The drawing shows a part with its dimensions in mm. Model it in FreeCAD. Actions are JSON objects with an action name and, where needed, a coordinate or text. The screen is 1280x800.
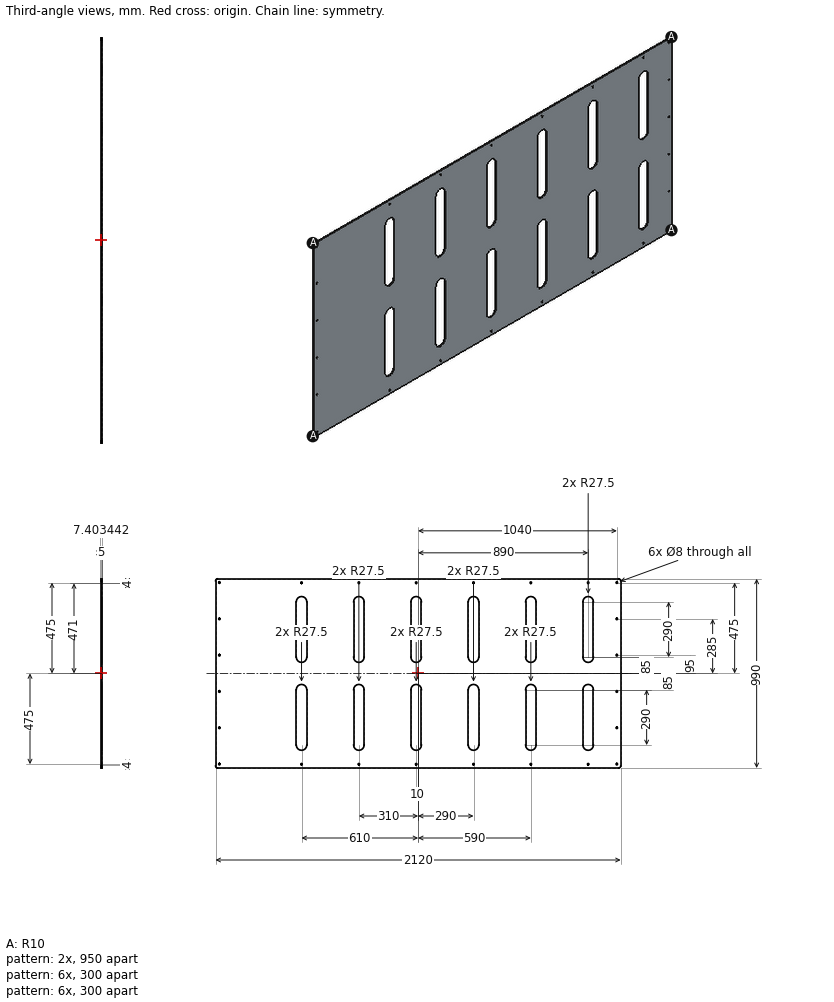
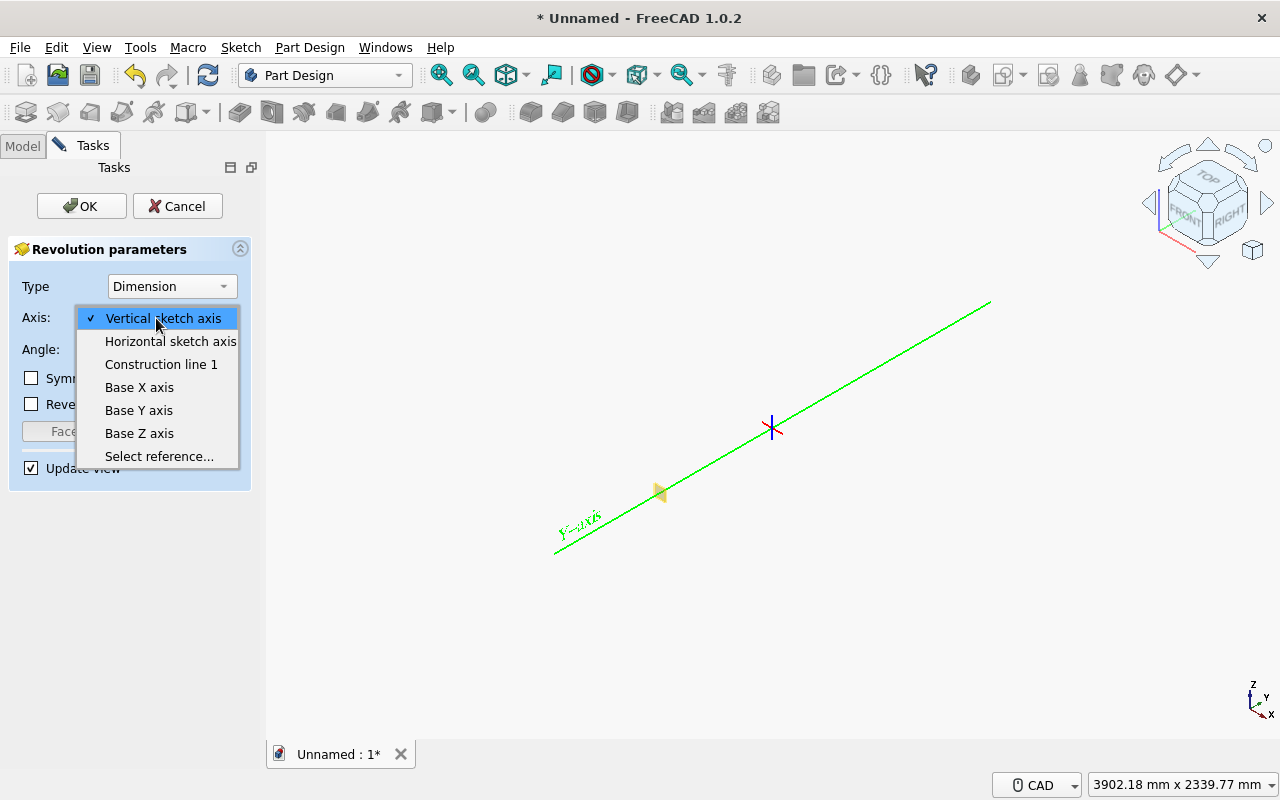
{"action": "left_click", "coordinate": [156, 364]}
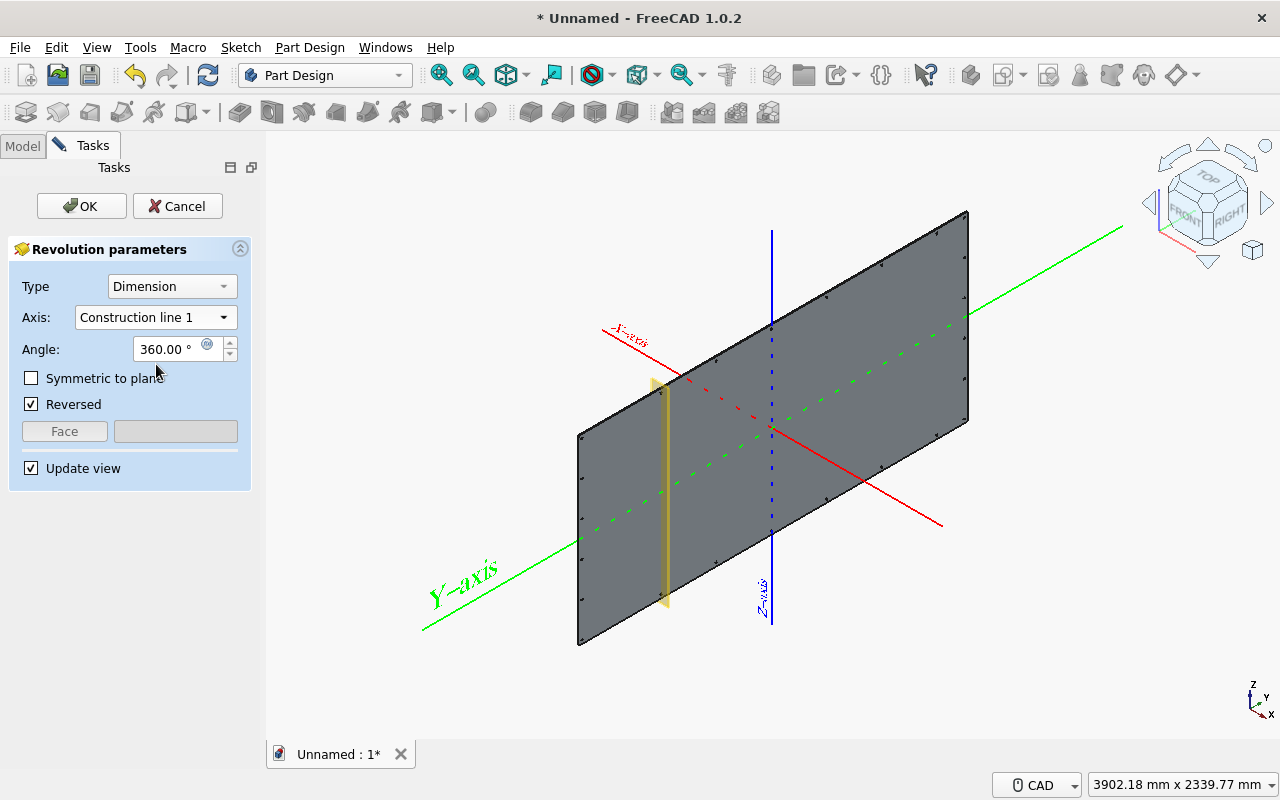
{"action": "left_click", "coordinate": [82, 206]}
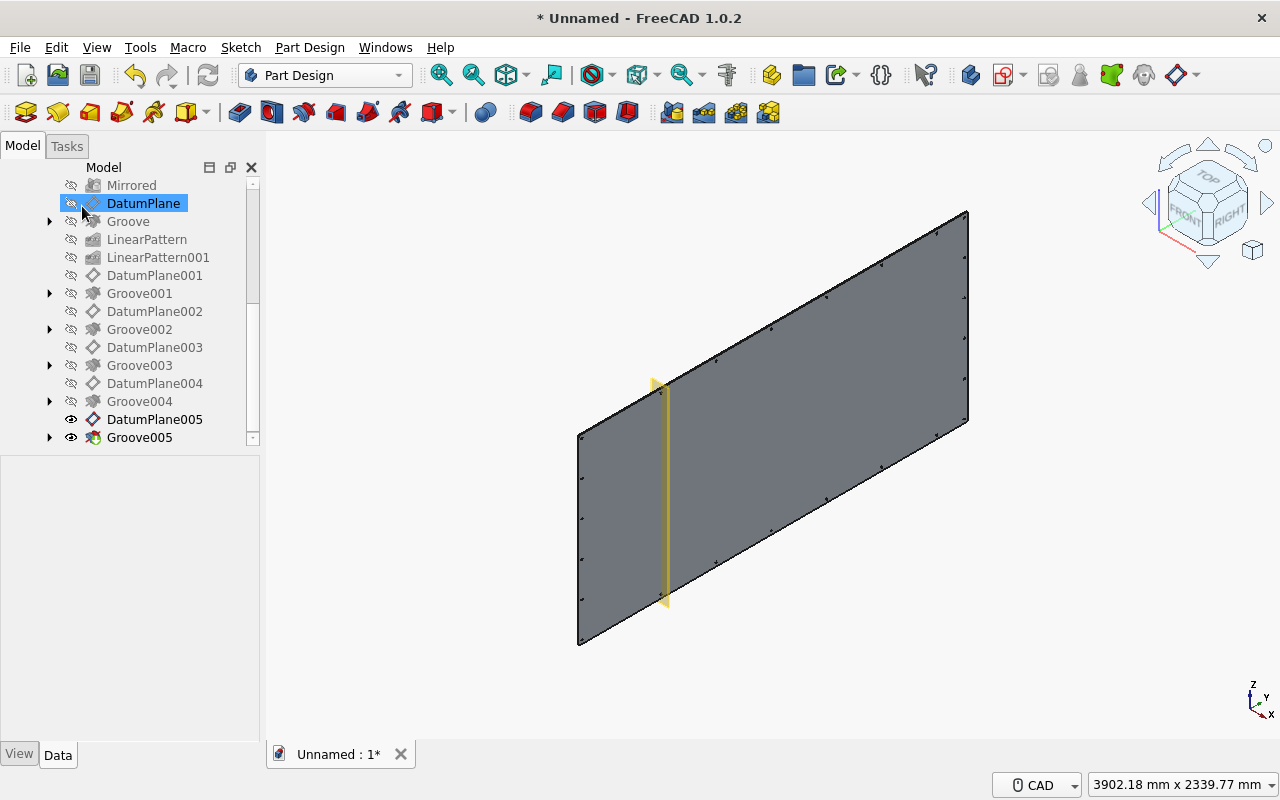
{"action": "left_click", "coordinate": [116, 419]}
{"action": "key", "text": "space"}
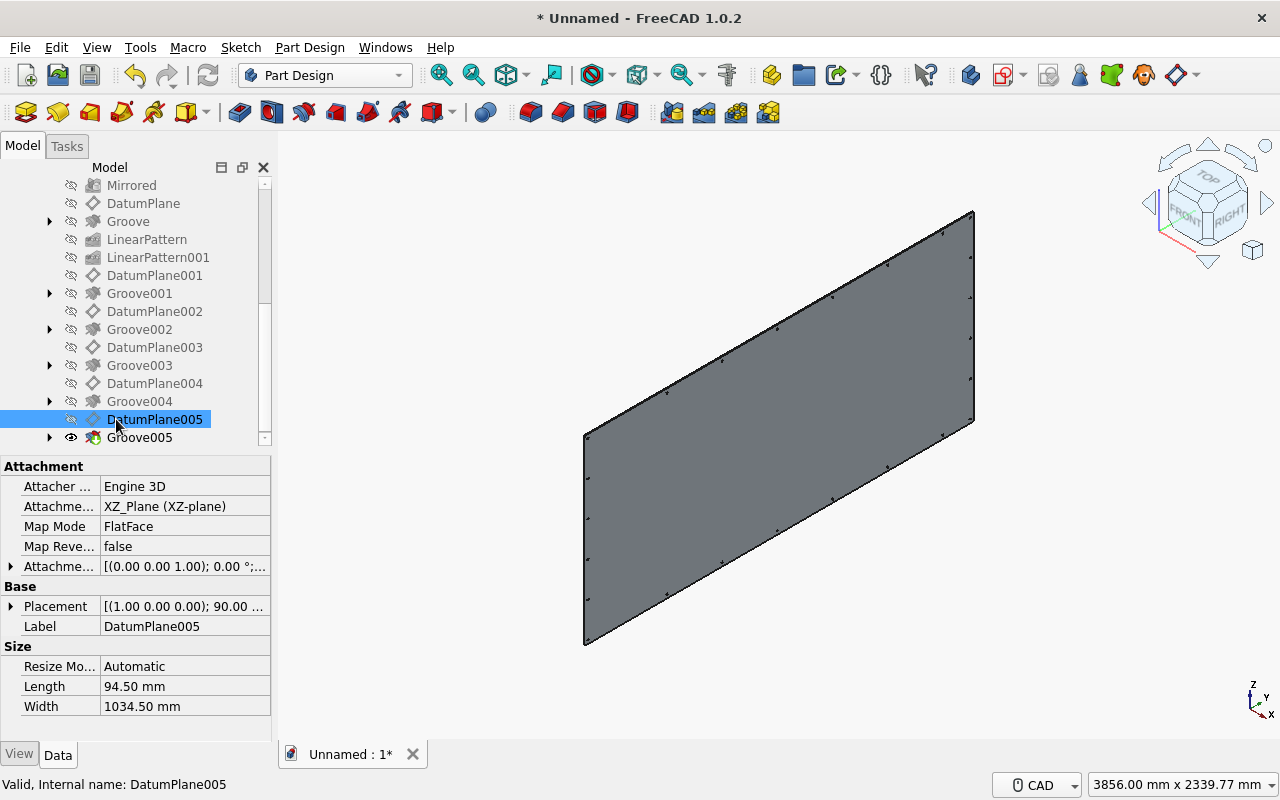
{"action": "left_click", "coordinate": [835, 396]}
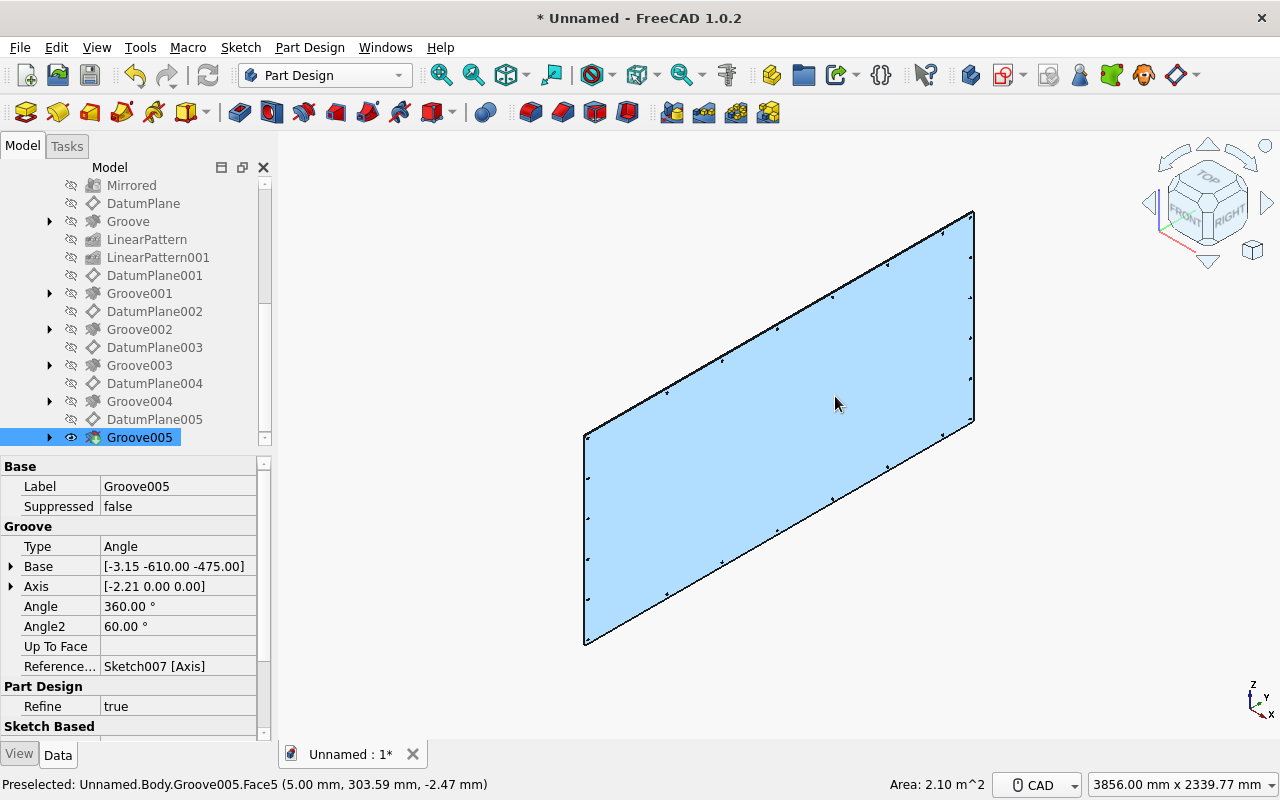
{"action": "left_click", "coordinate": [1004, 76]}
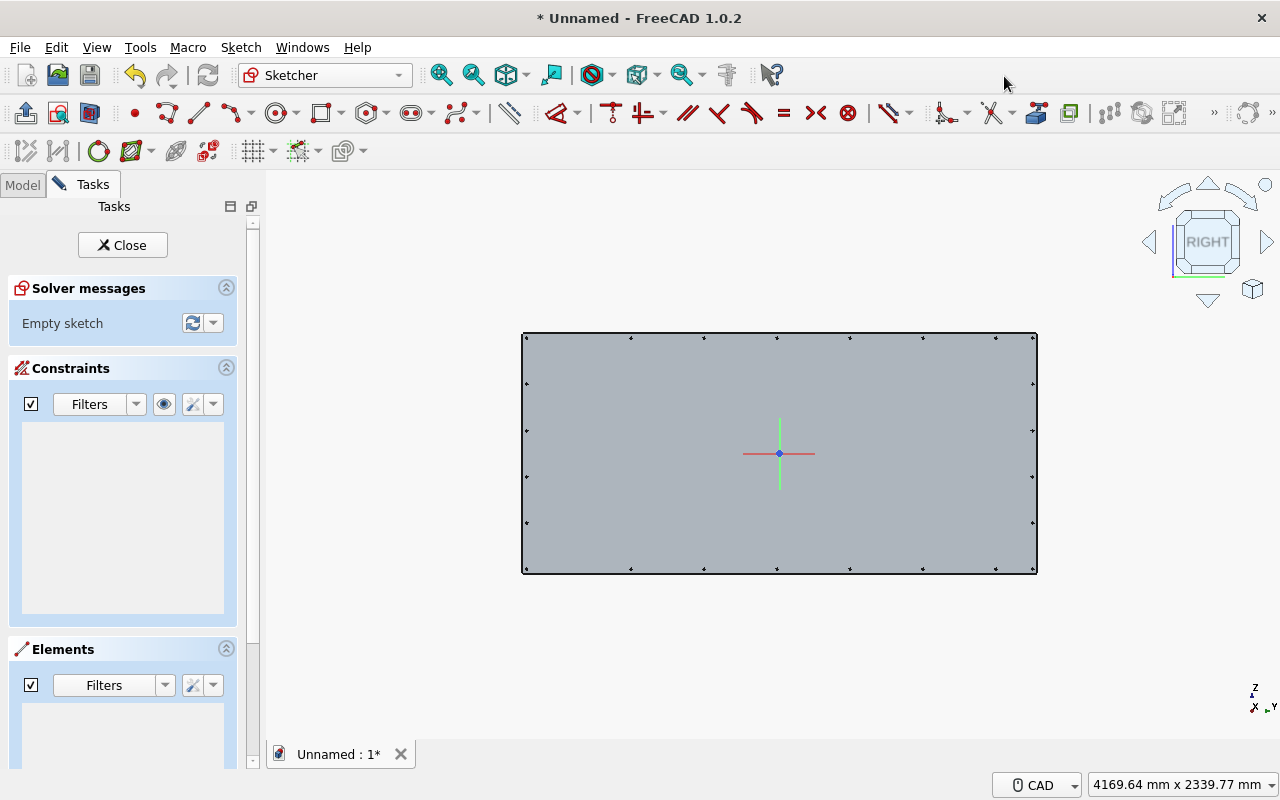
{"action": "scroll", "coordinate": [1091, 379], "scroll_direction": "up", "scroll_amount": 7}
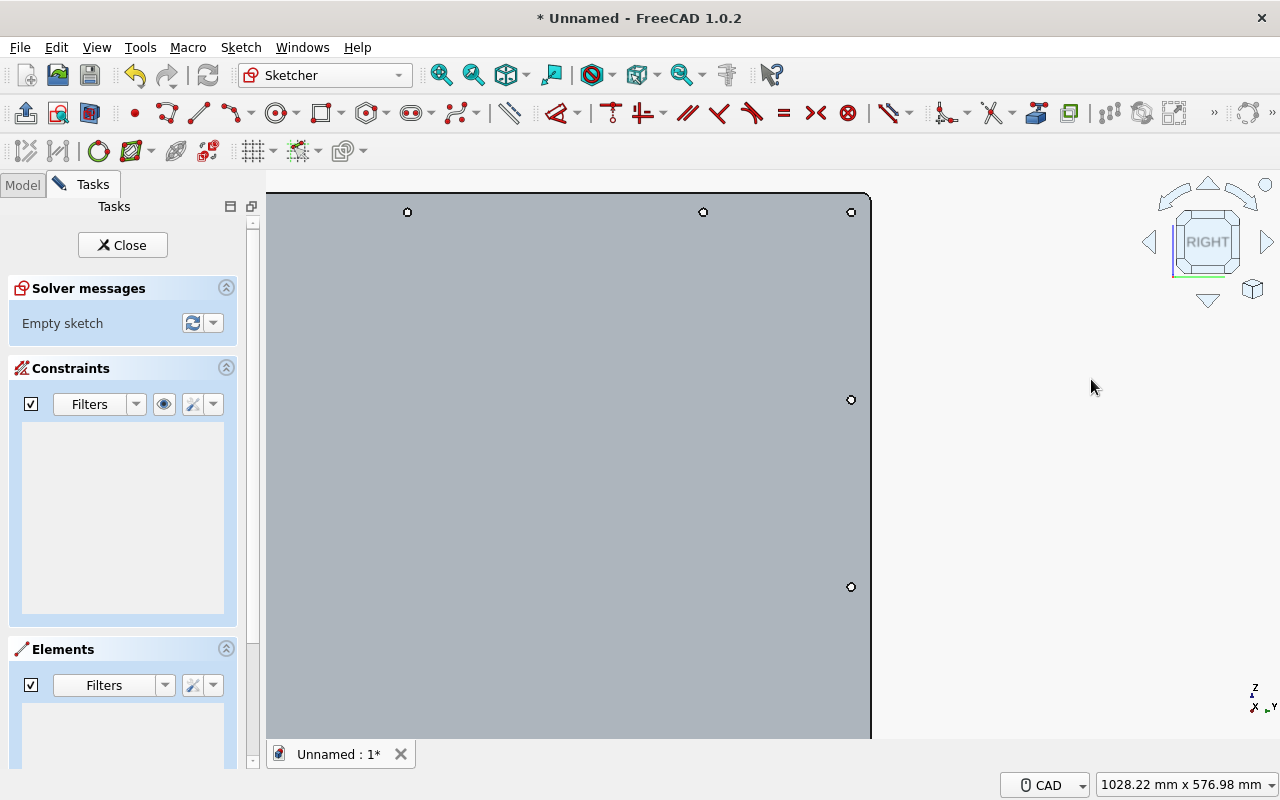
{"action": "left_click", "coordinate": [412, 114]}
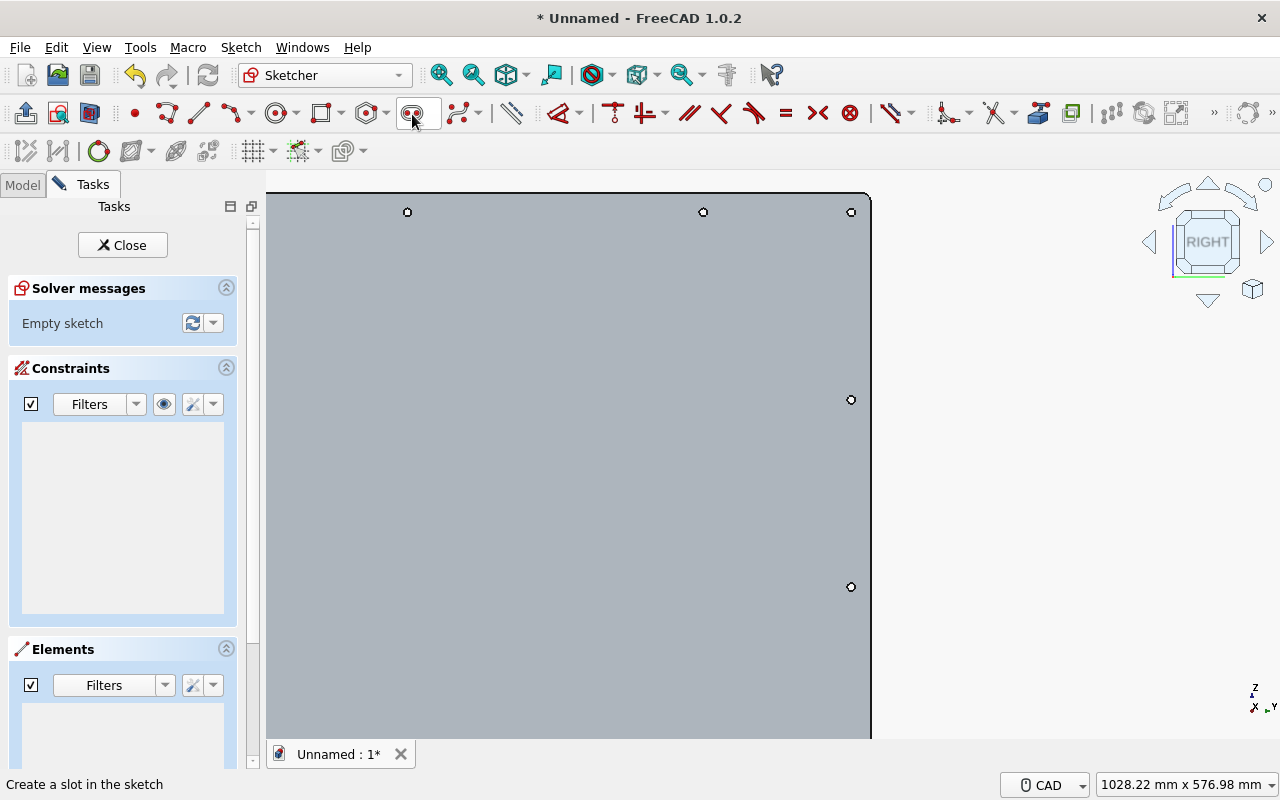
{"action": "left_click", "coordinate": [703, 597]}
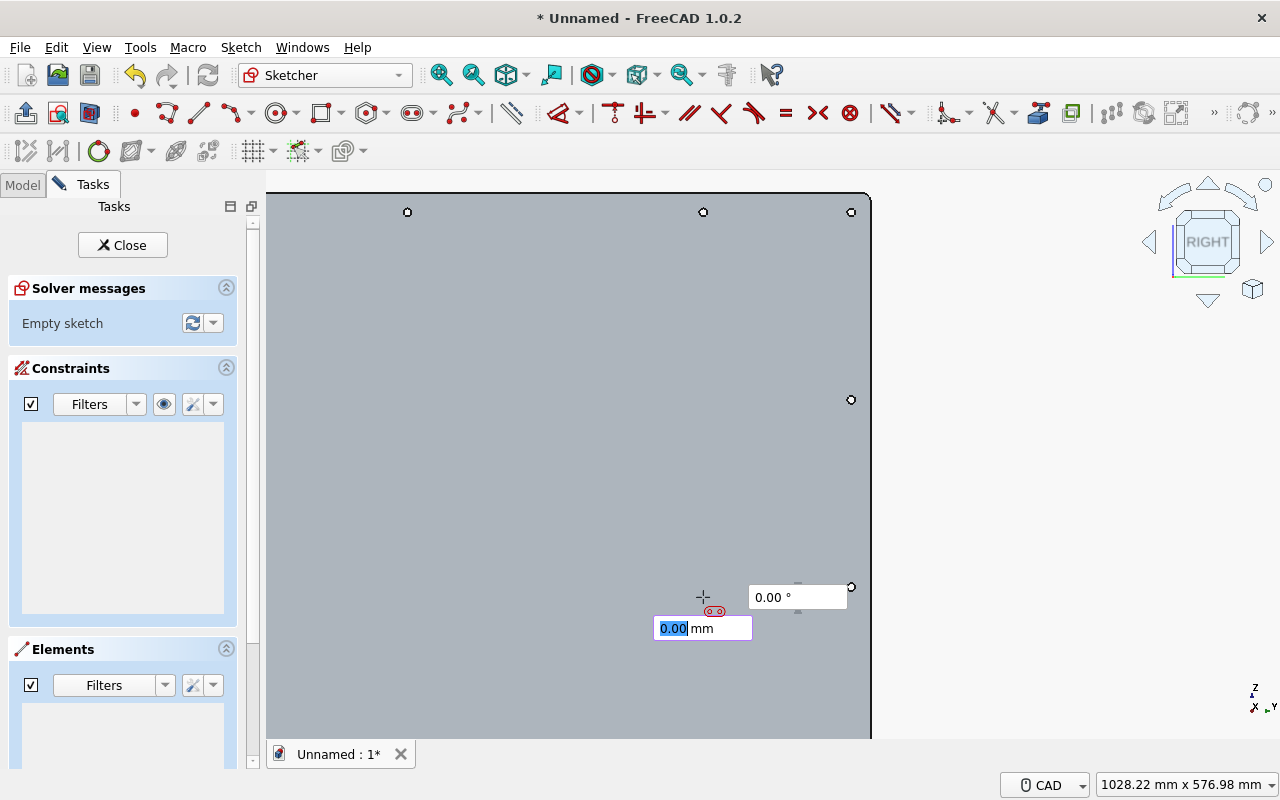
{"action": "left_click", "coordinate": [703, 311]}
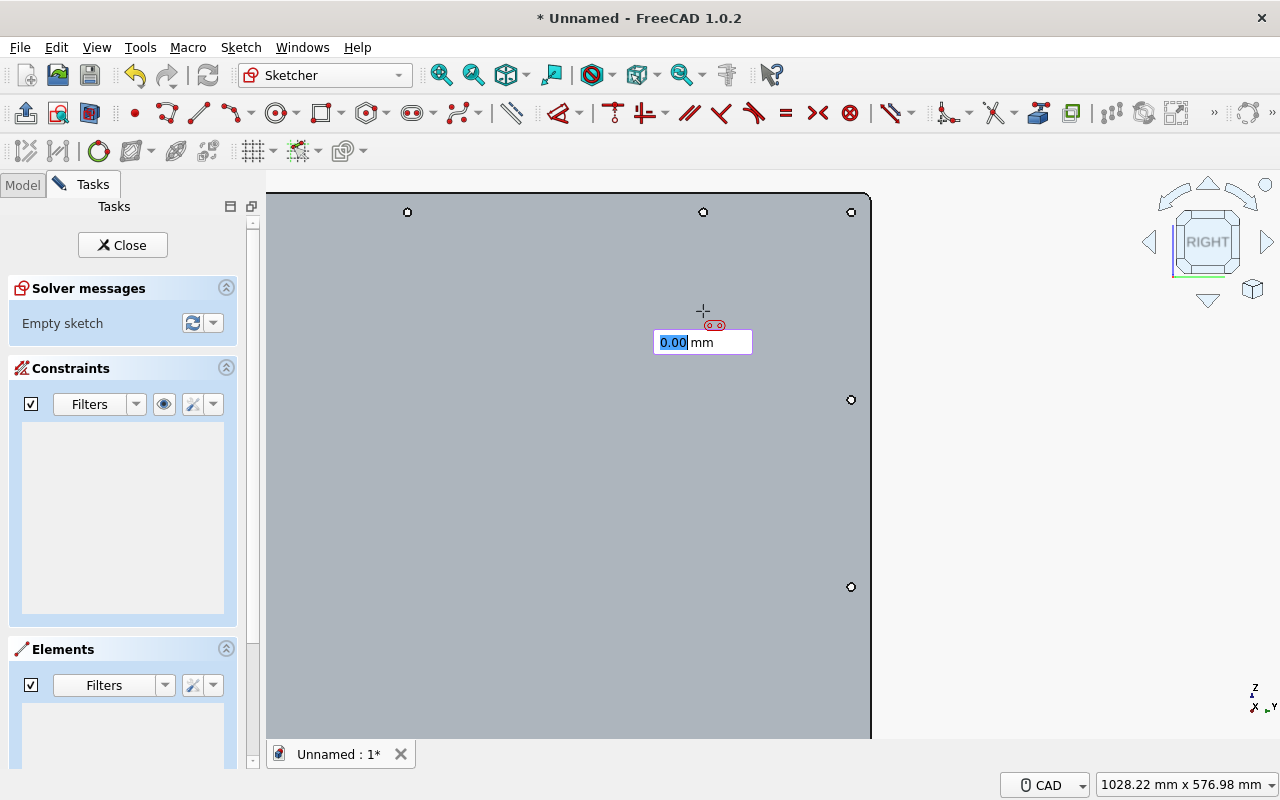
{"action": "left_click", "coordinate": [731, 454]}
{"action": "key", "text": "Escape"}